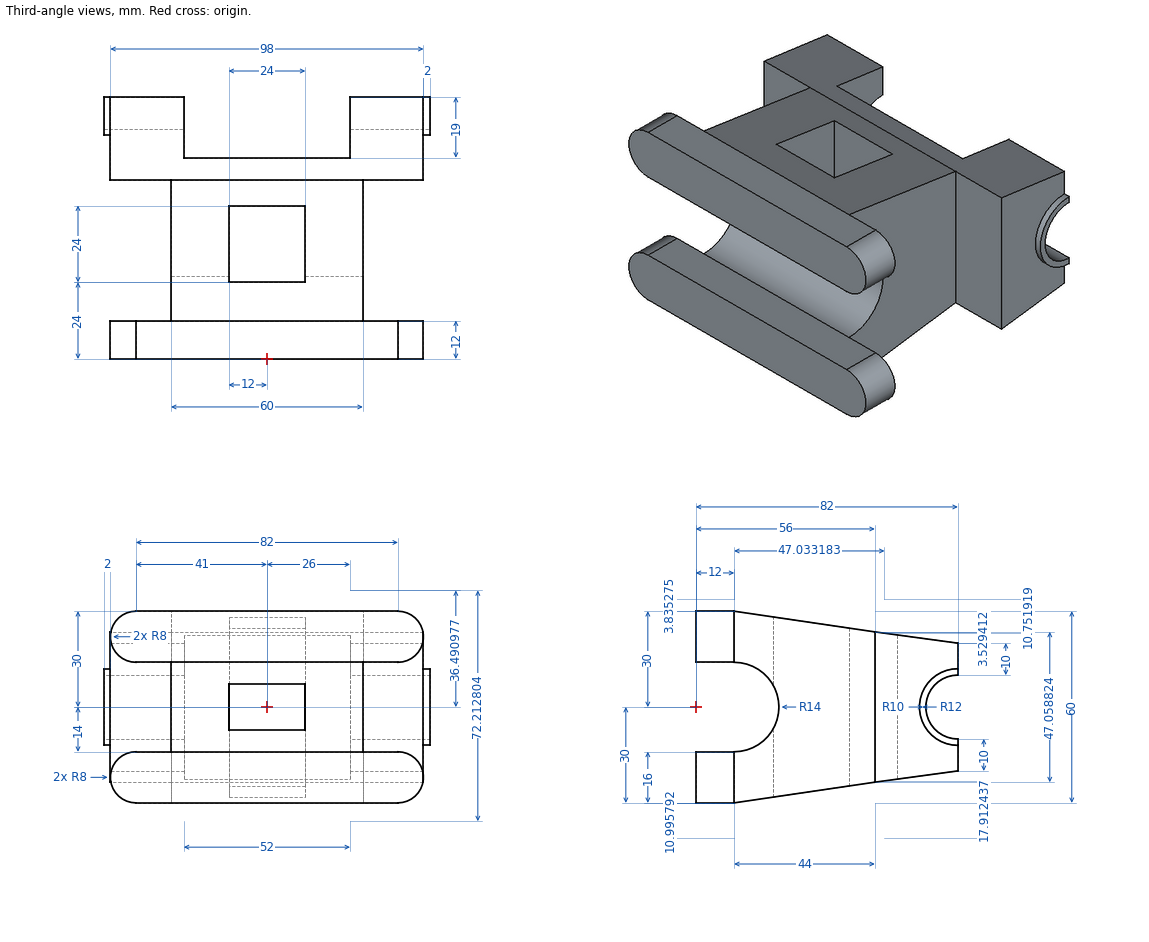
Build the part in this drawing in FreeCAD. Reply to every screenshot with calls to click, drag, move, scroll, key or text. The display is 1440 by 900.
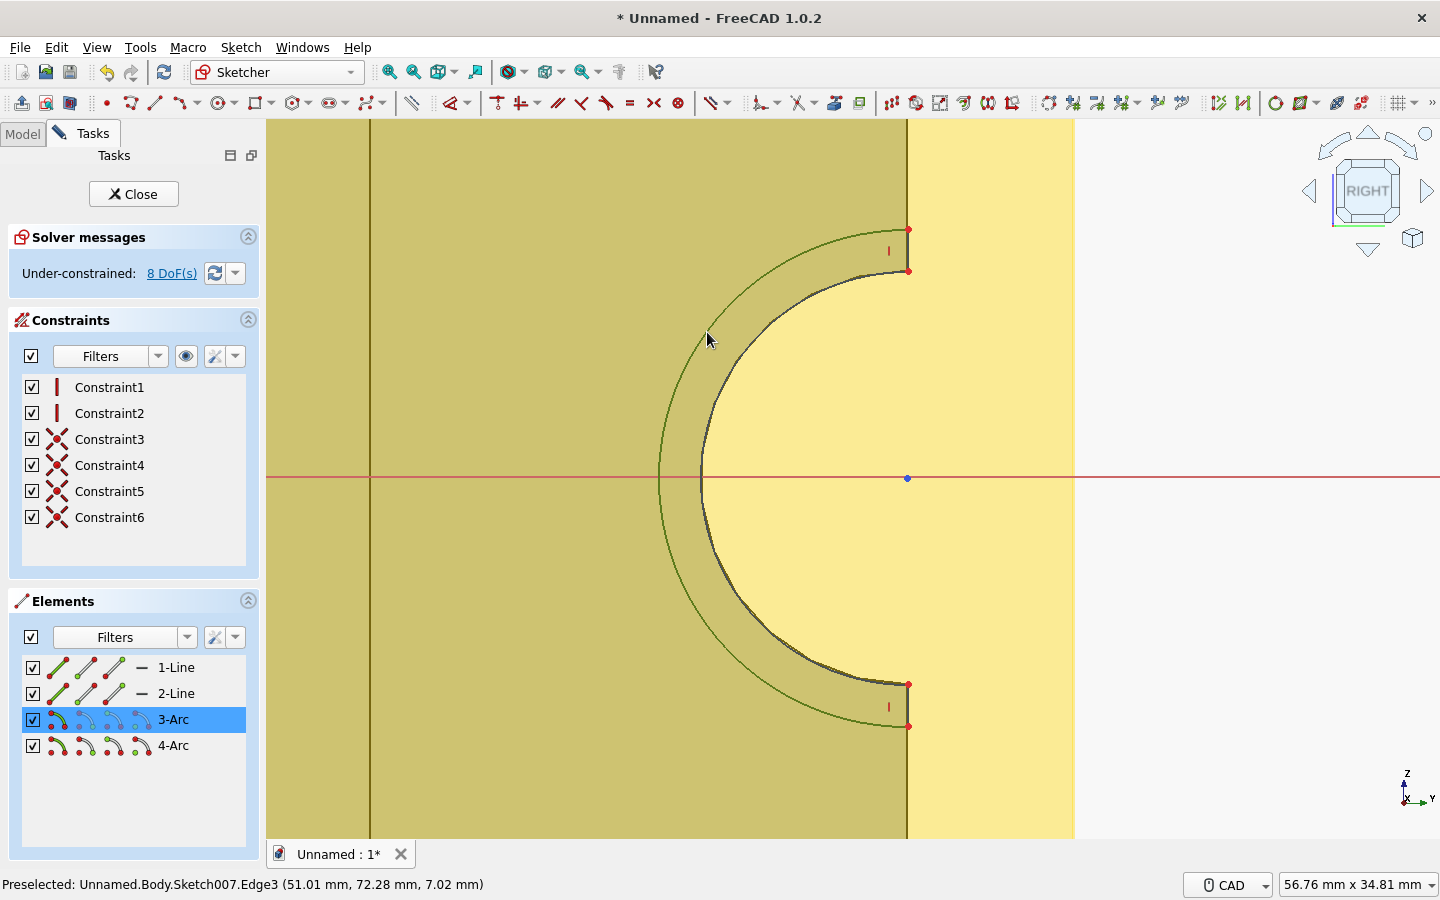
click(741, 357)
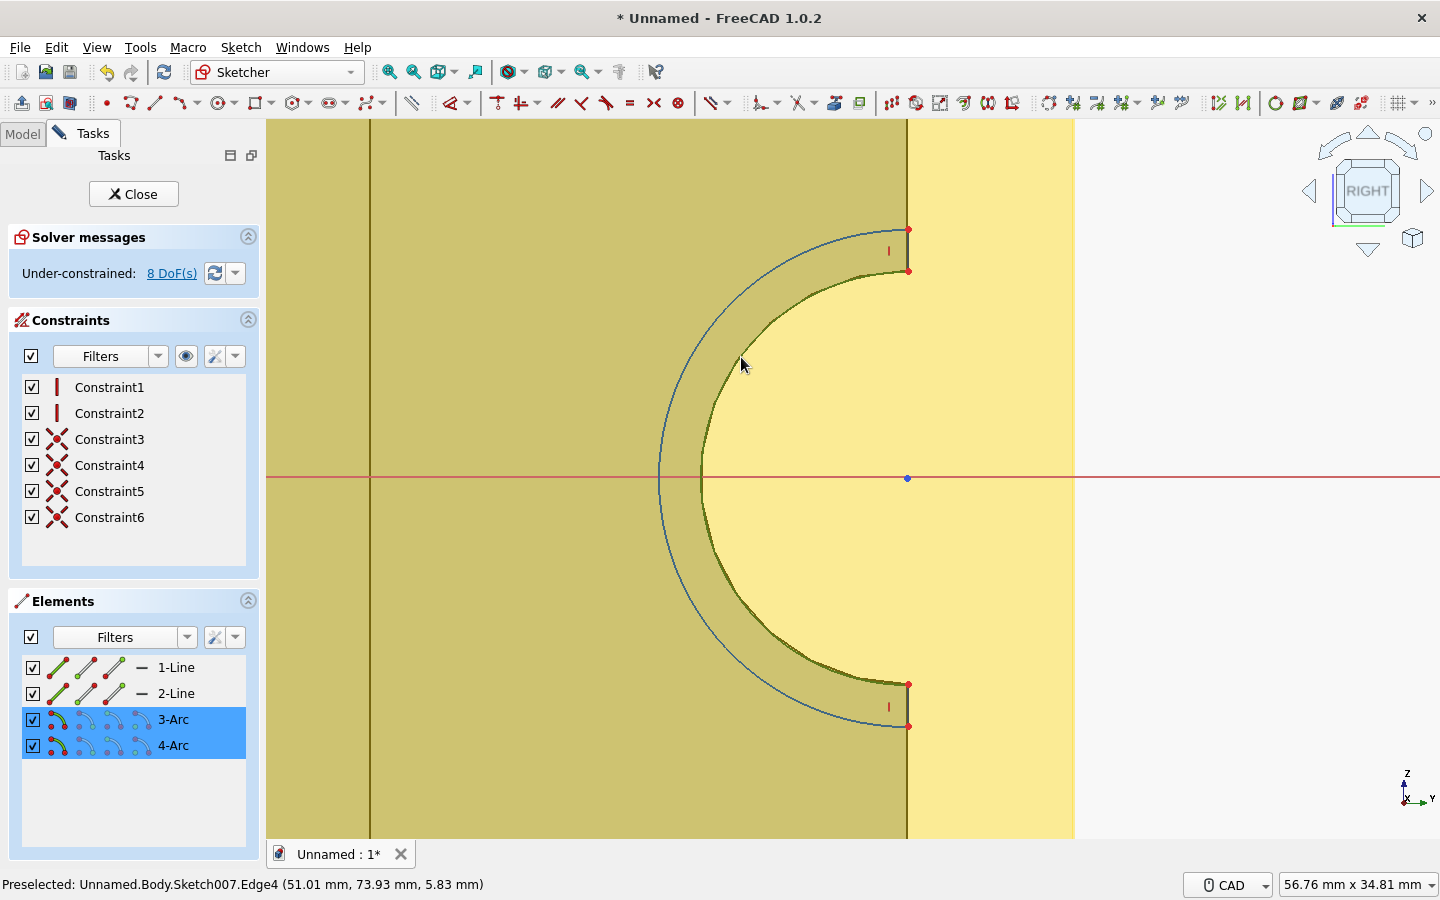
click(498, 104)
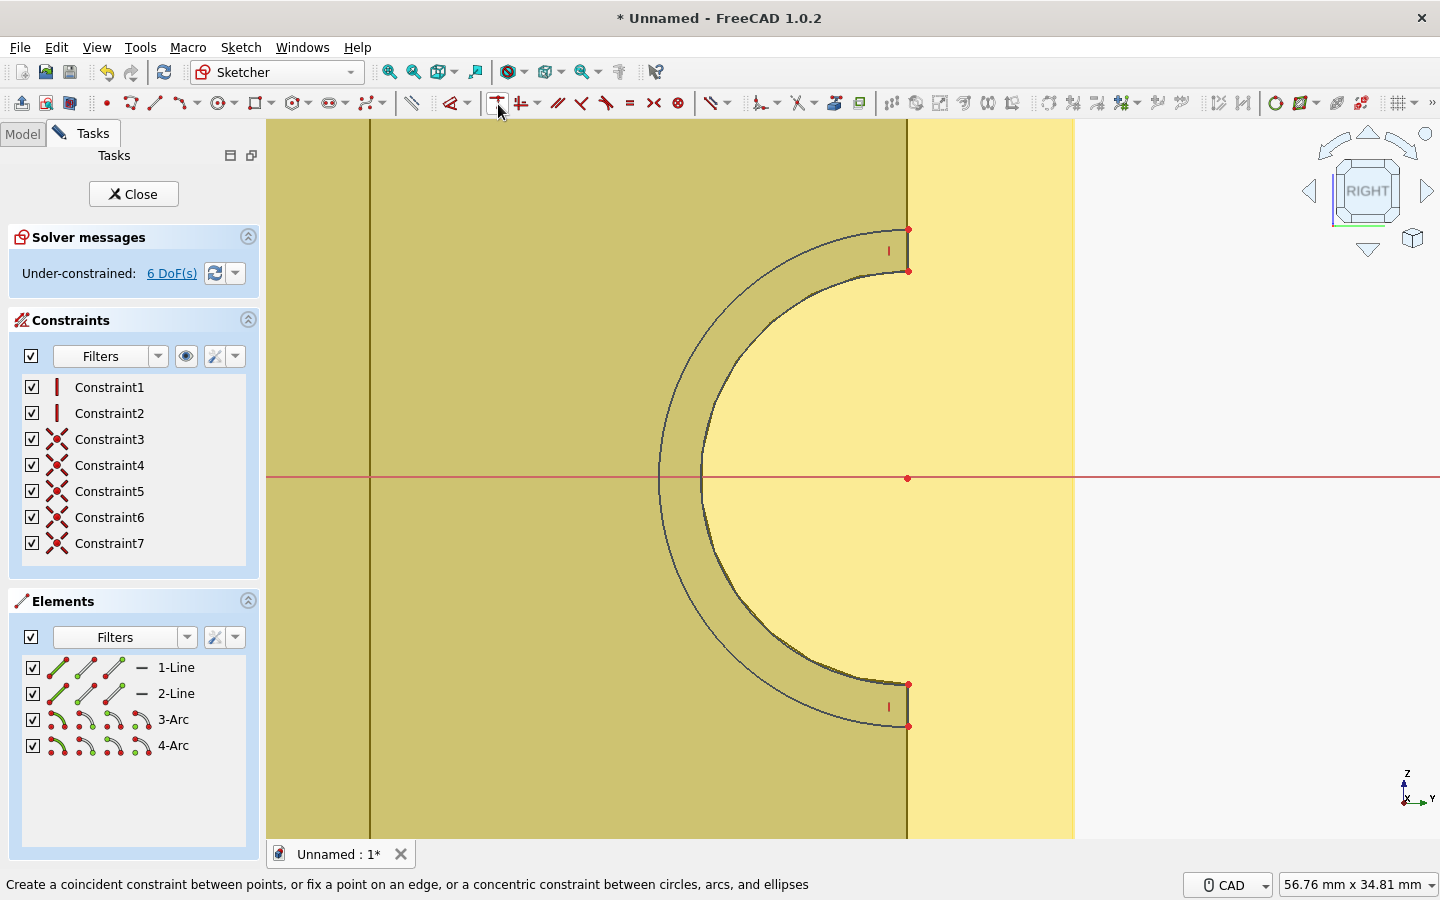
click(907, 479)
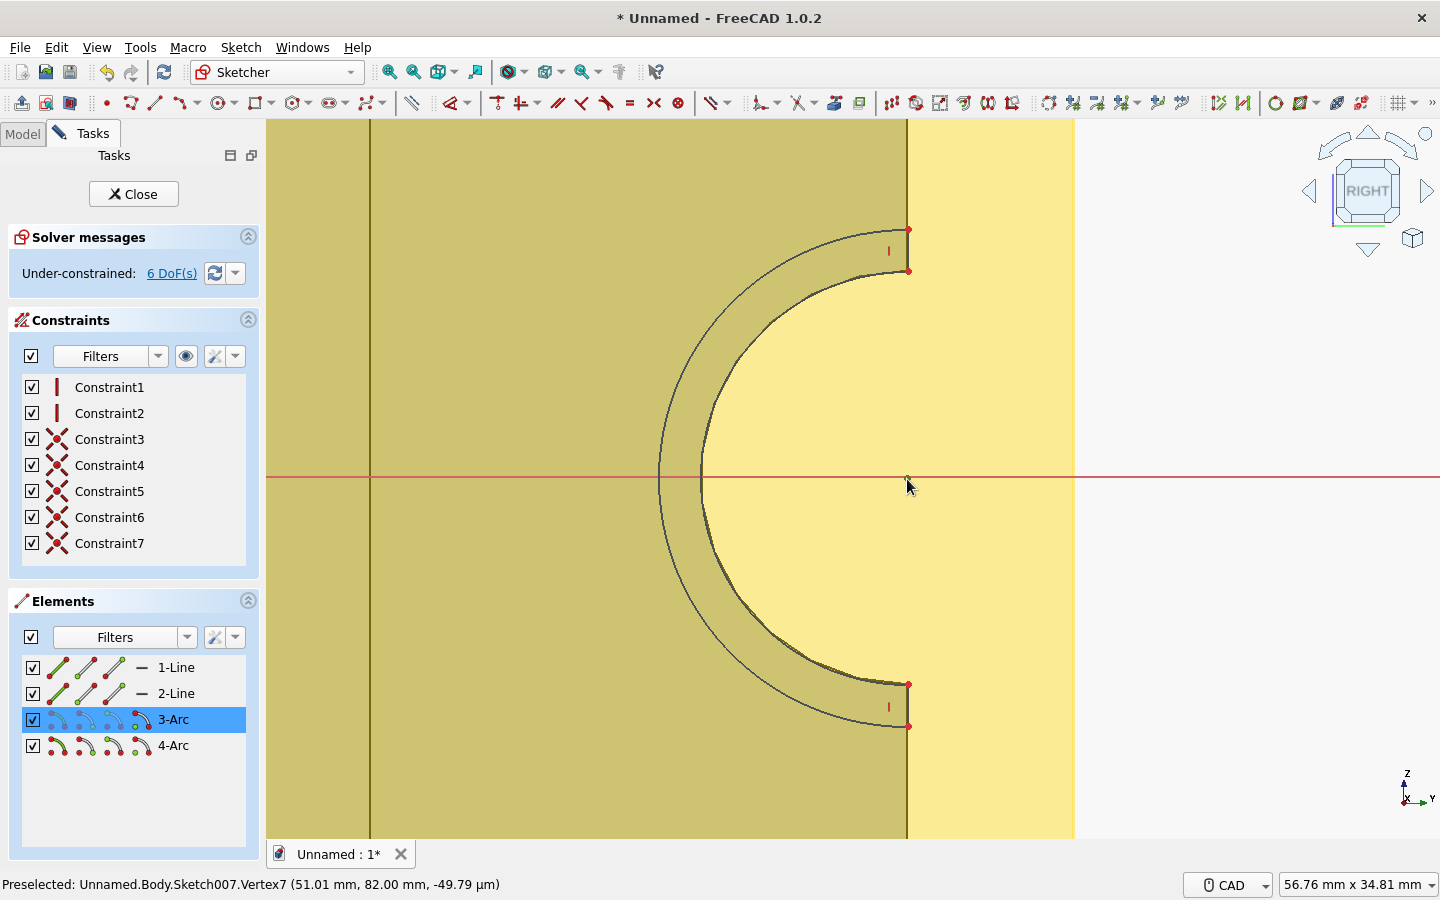
click(364, 477)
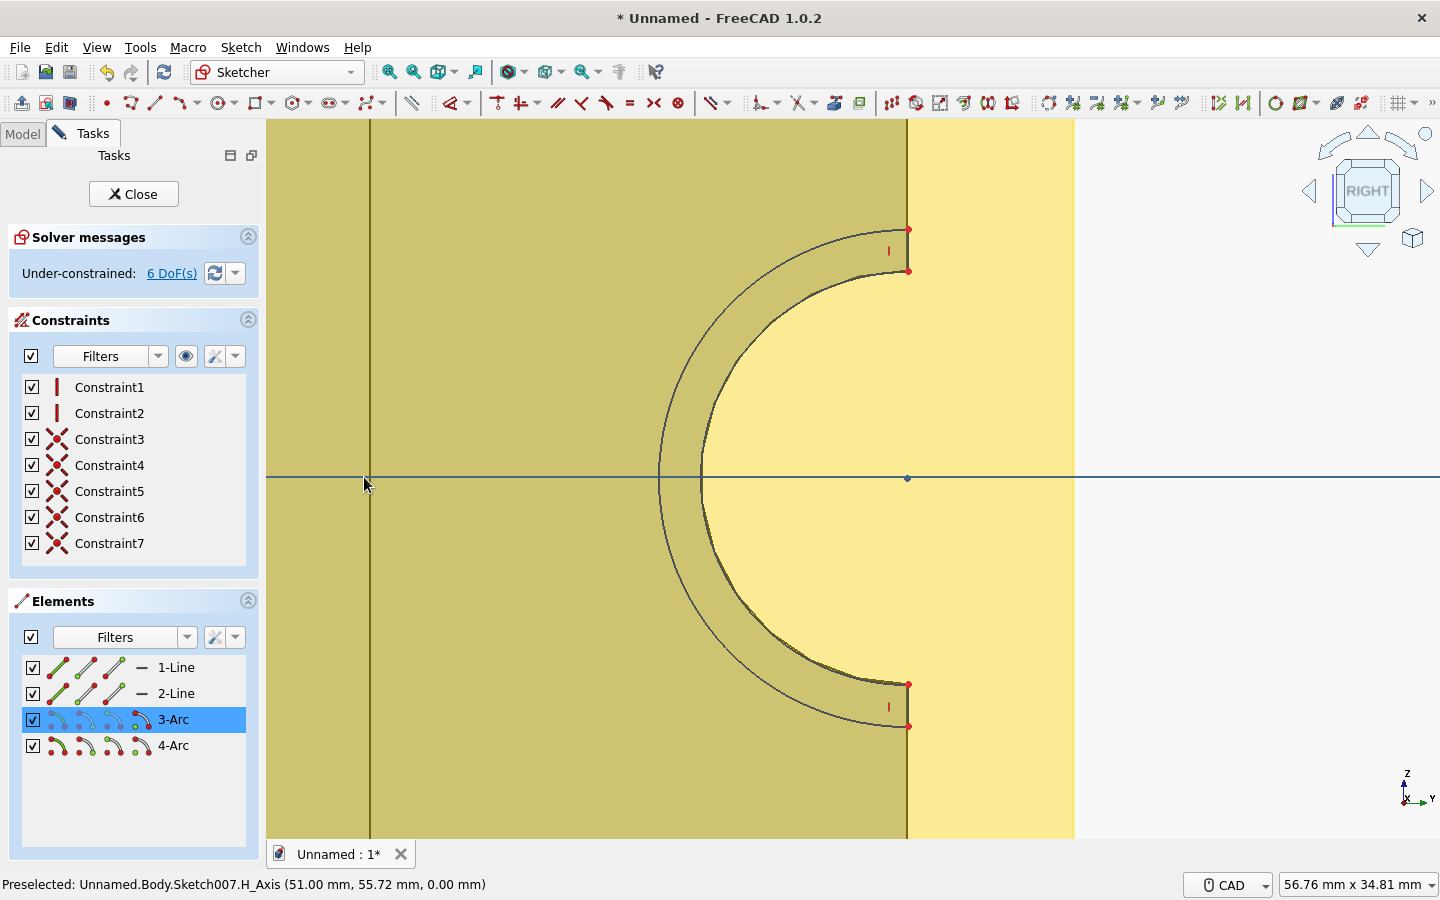
click(498, 104)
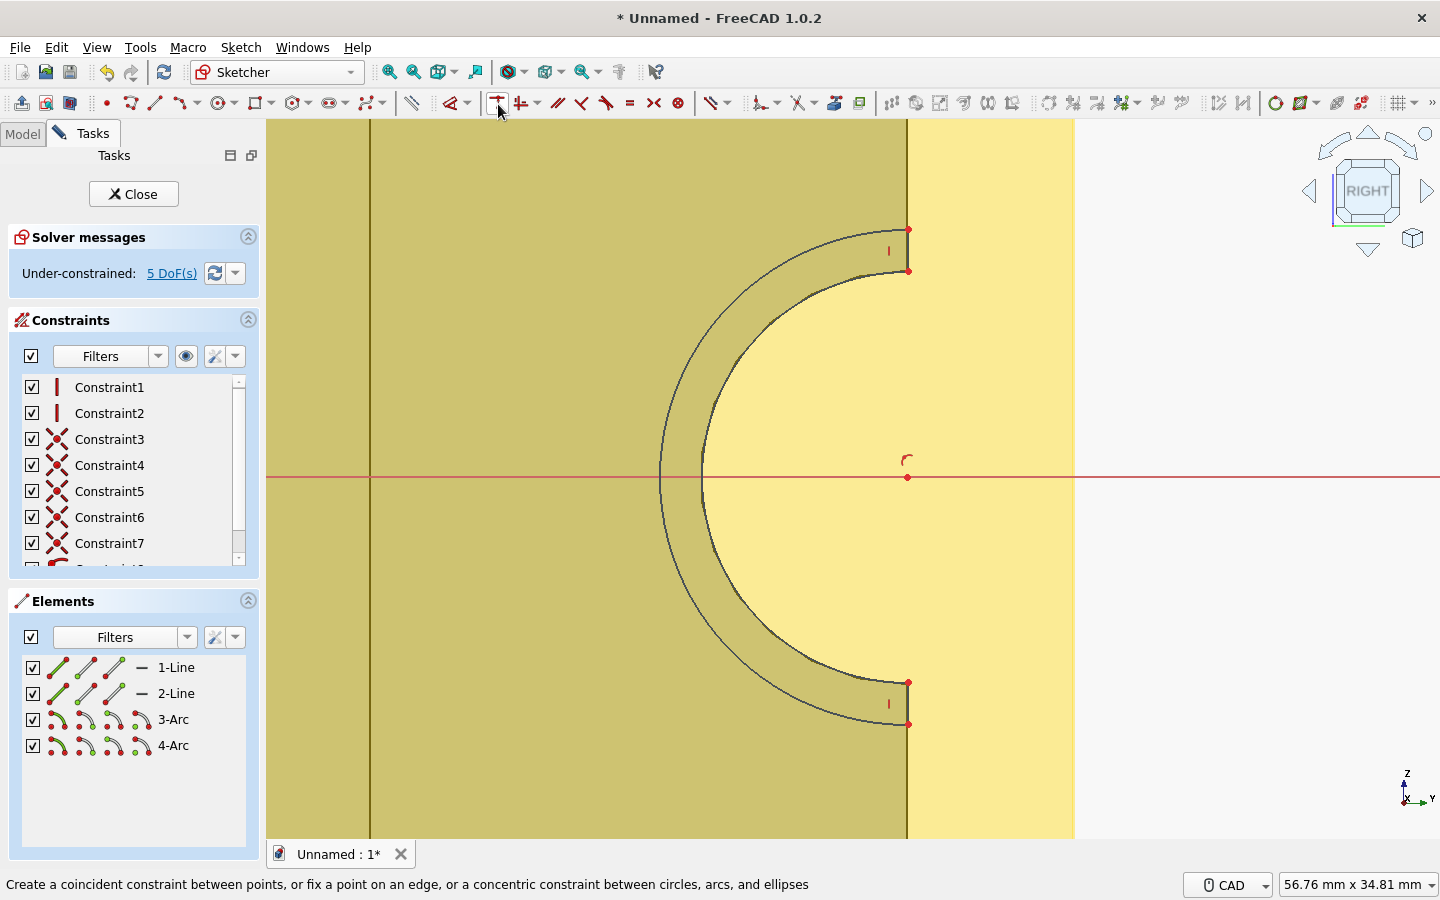
click(450, 104)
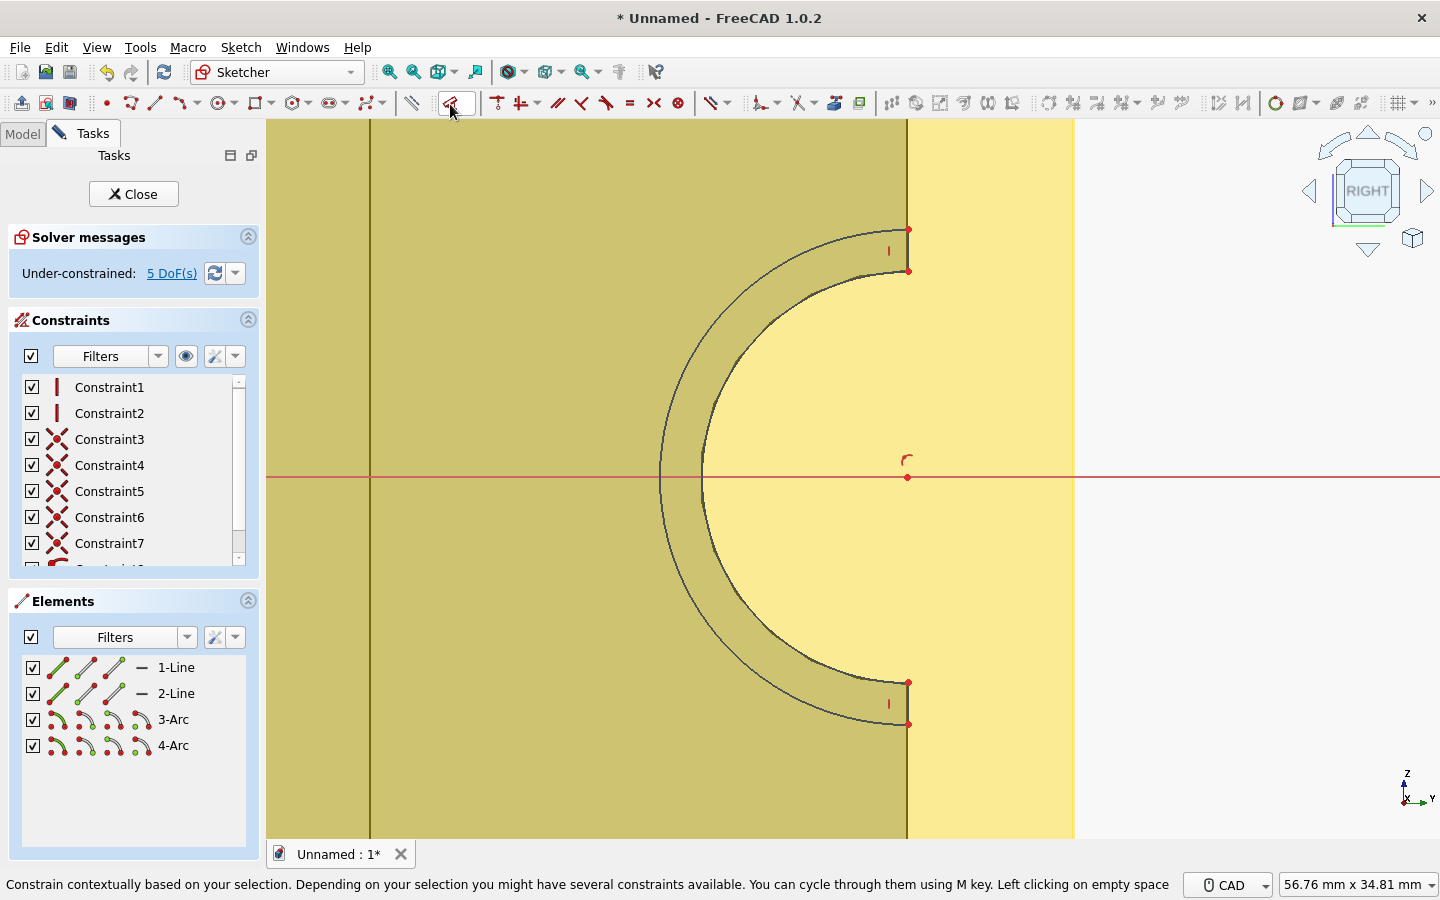
click(707, 332)
click(681, 313)